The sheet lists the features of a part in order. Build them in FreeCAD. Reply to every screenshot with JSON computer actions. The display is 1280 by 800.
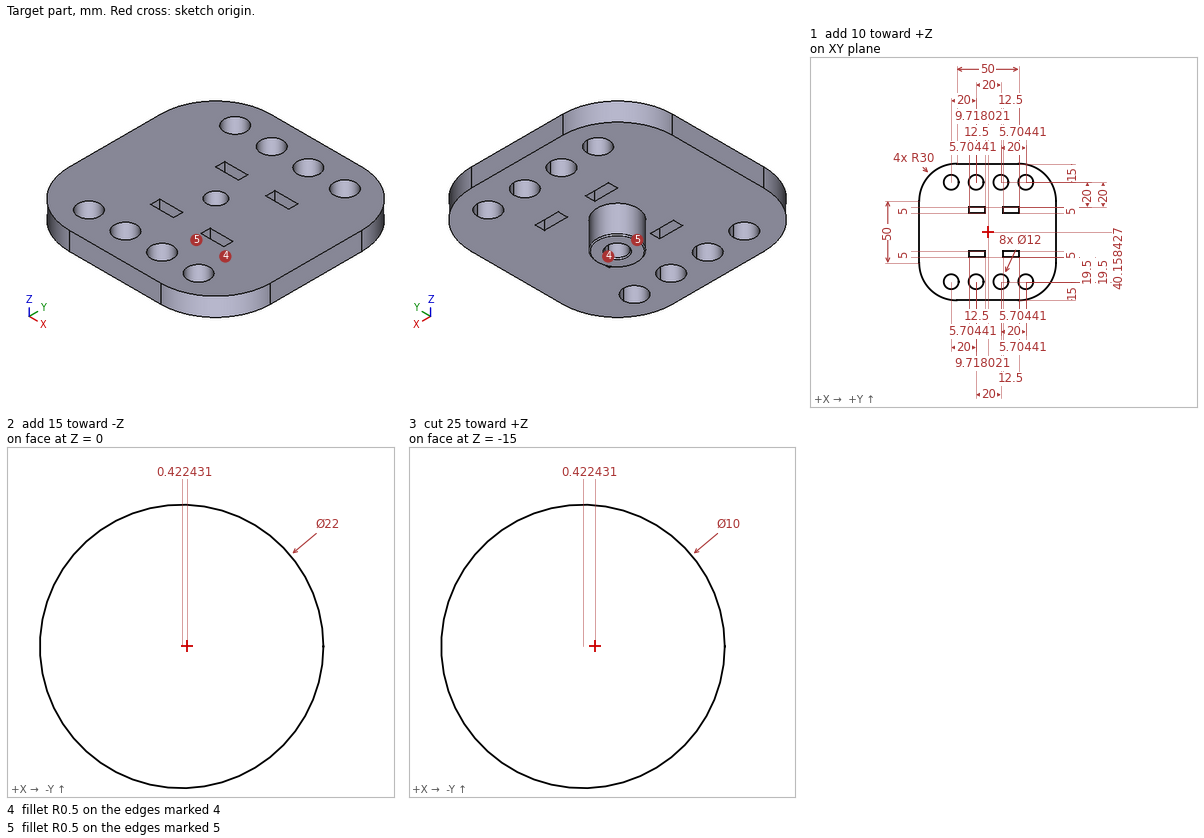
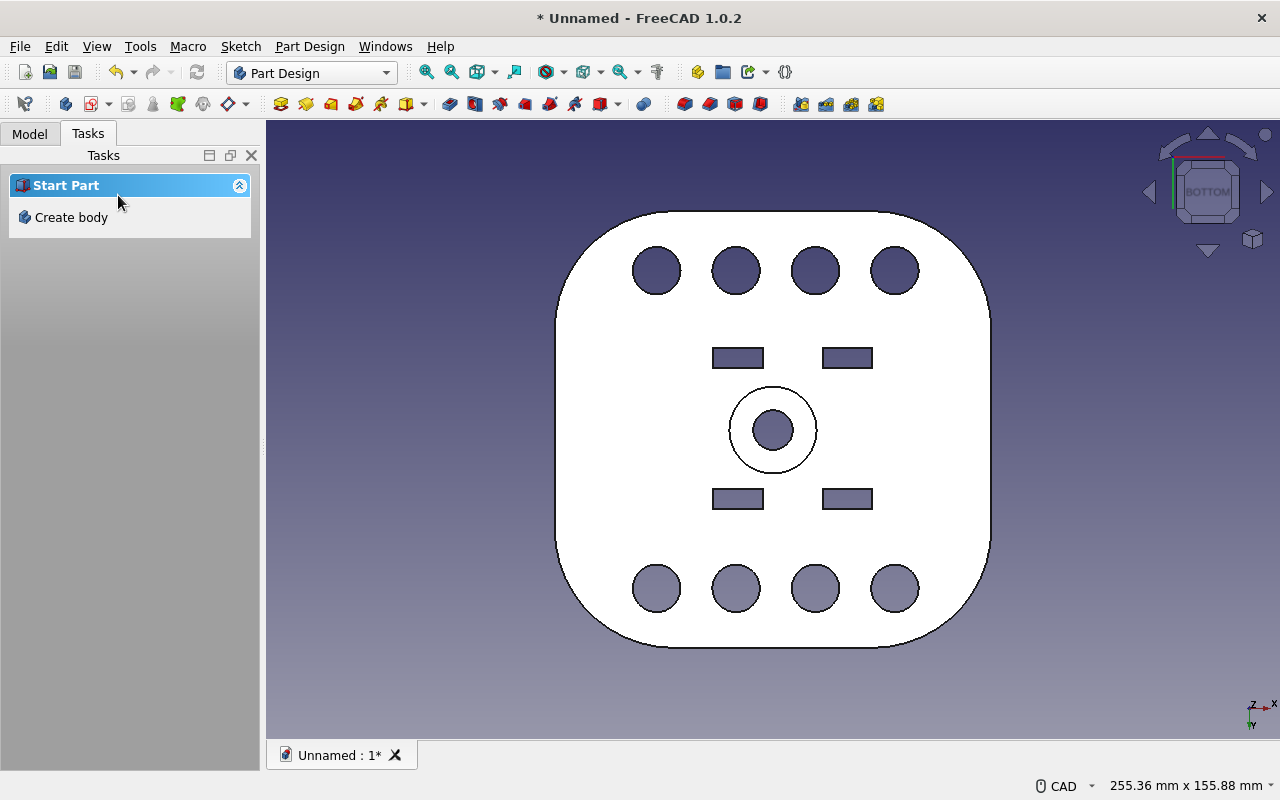
{"action": "left_click", "coordinate": [753, 429]}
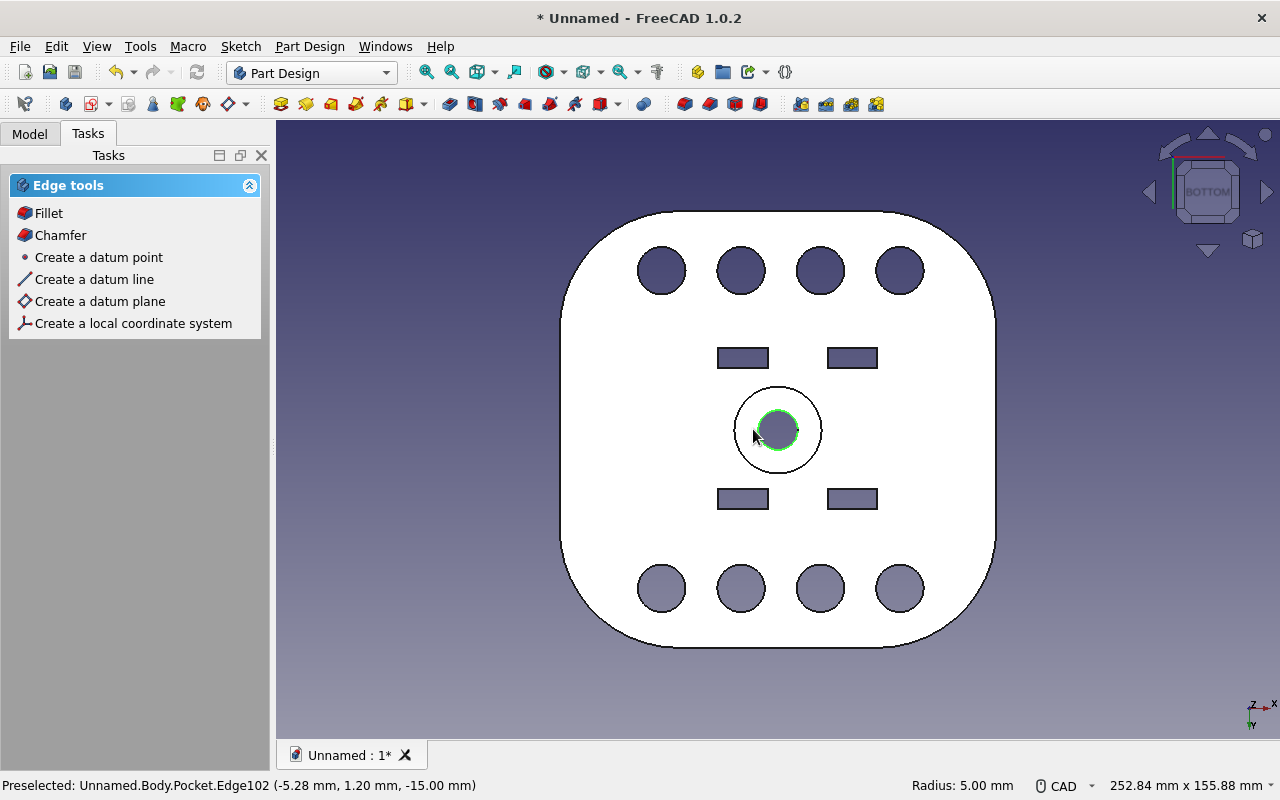
{"action": "left_click", "coordinate": [685, 104]}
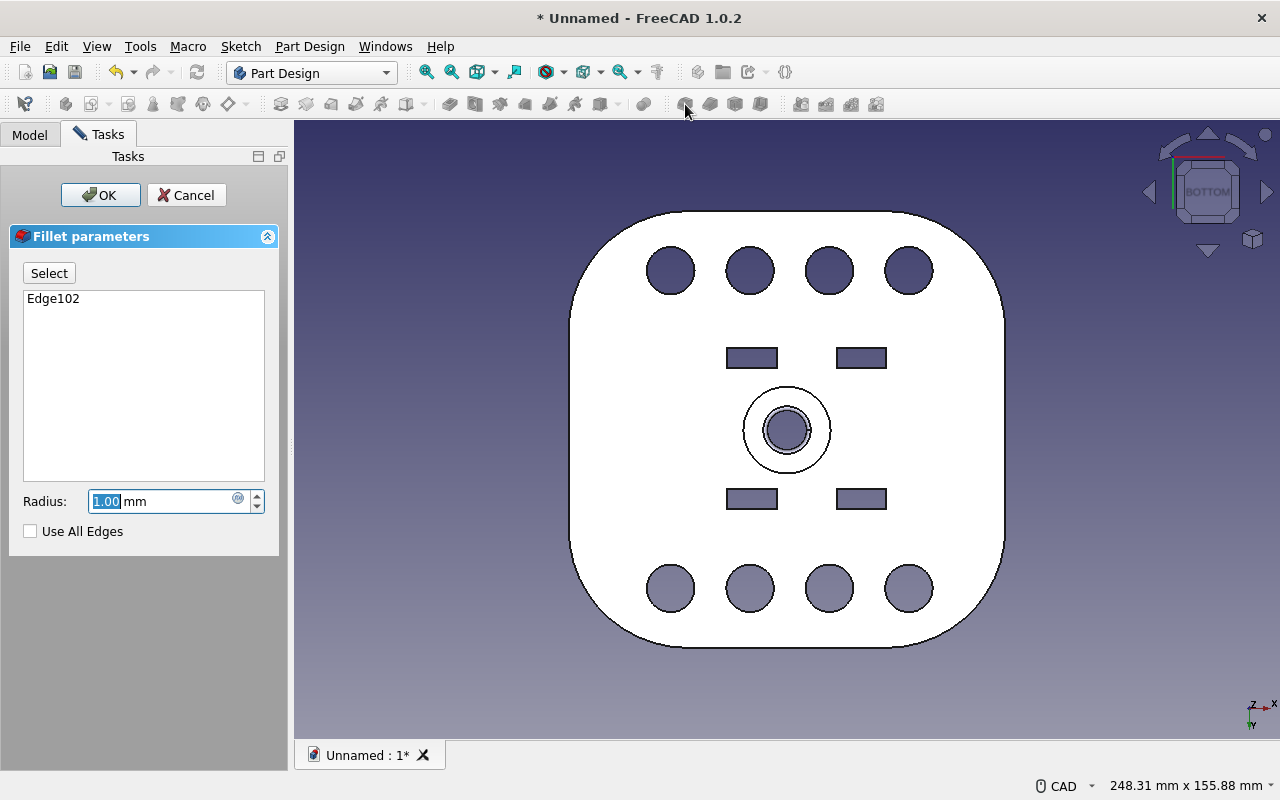
{"action": "type", "text": "0.5"}
{"action": "key", "text": "Tab"}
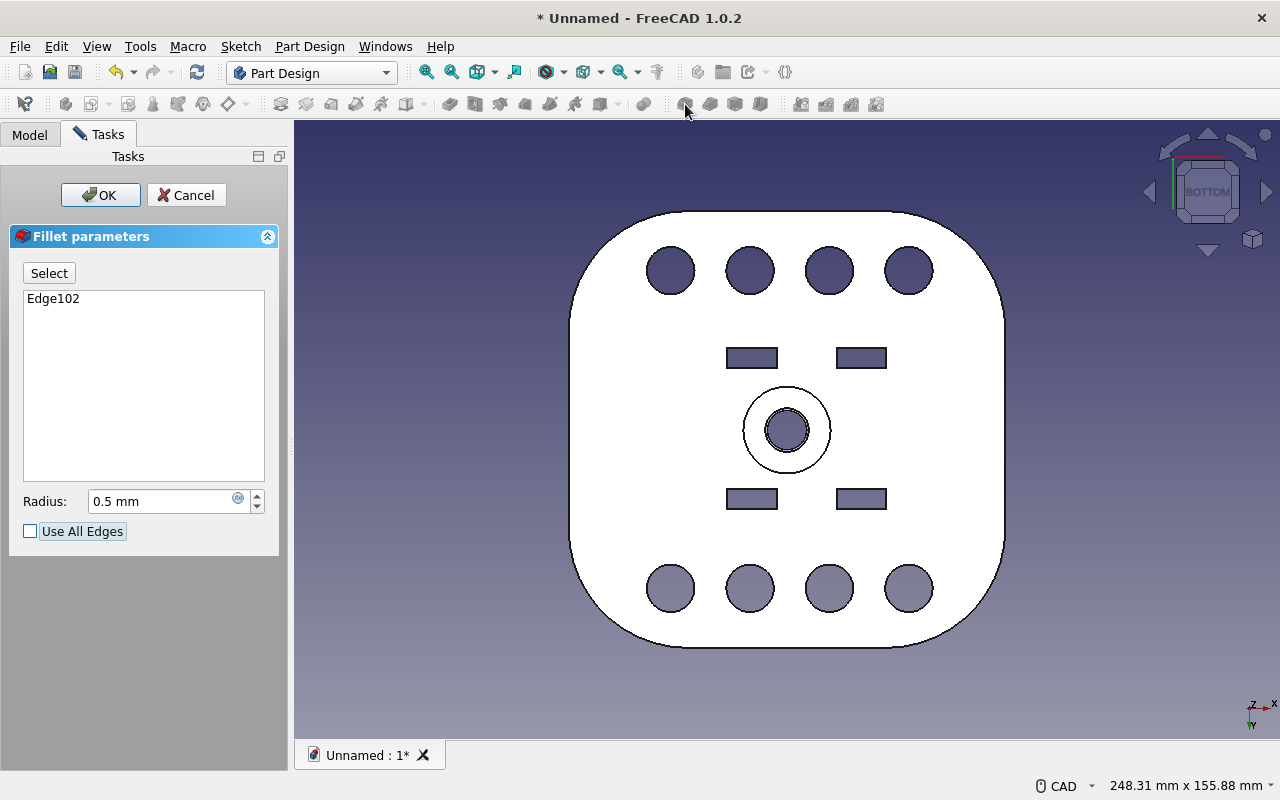
{"action": "left_click", "coordinate": [101, 195]}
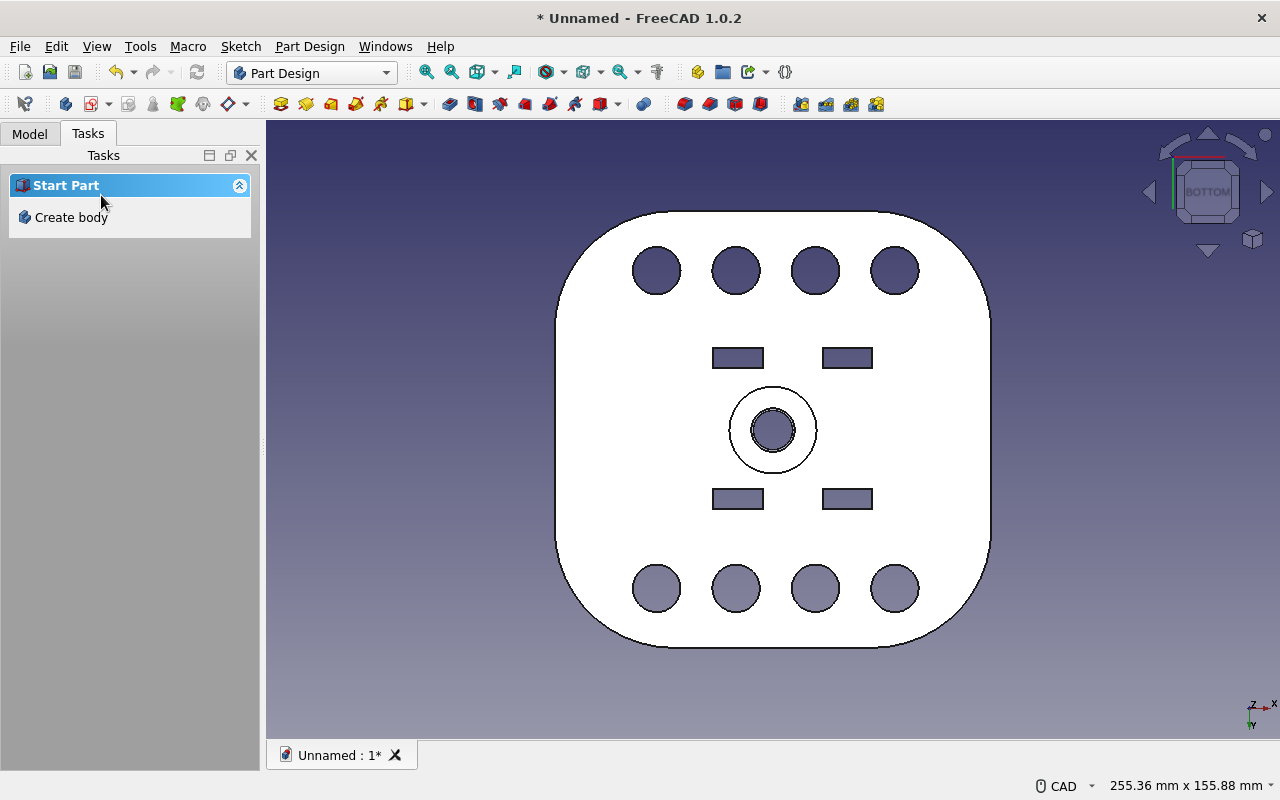
{"action": "left_click", "coordinate": [729, 429]}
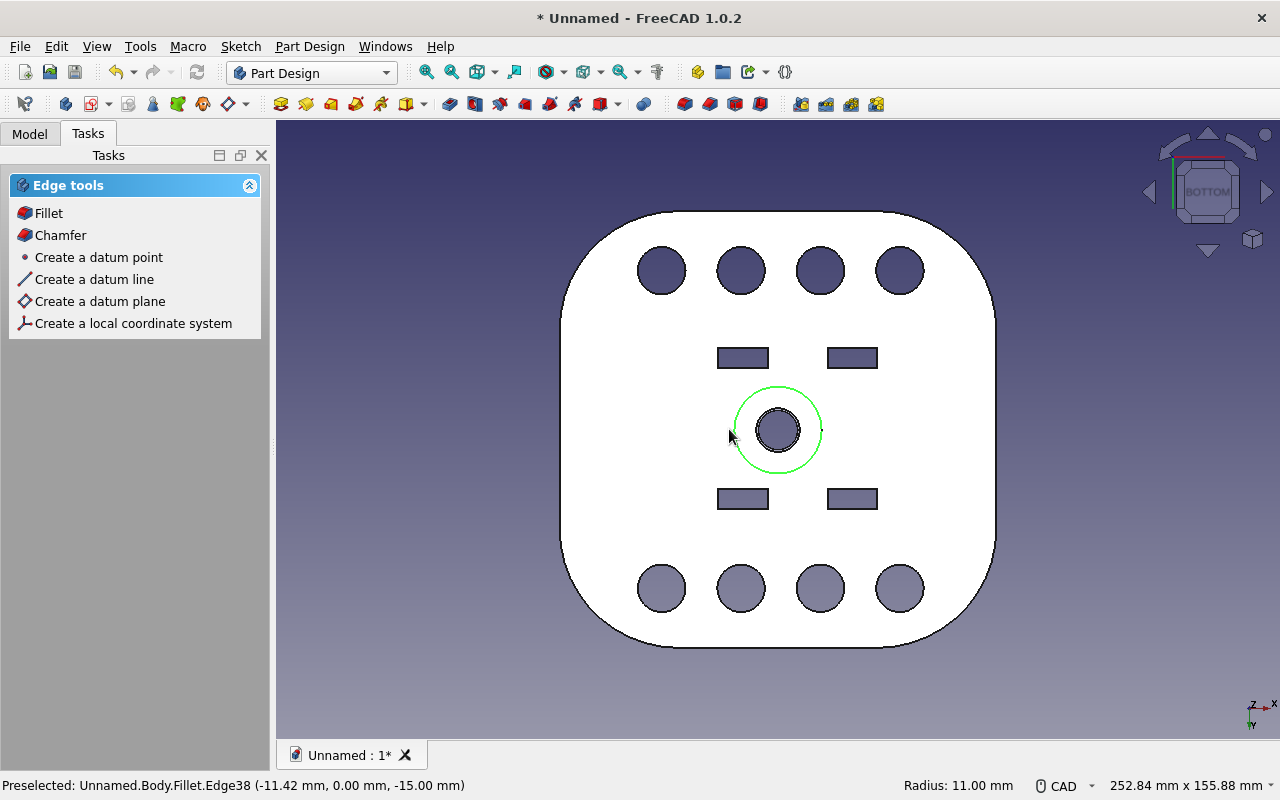
{"action": "left_click", "coordinate": [685, 104]}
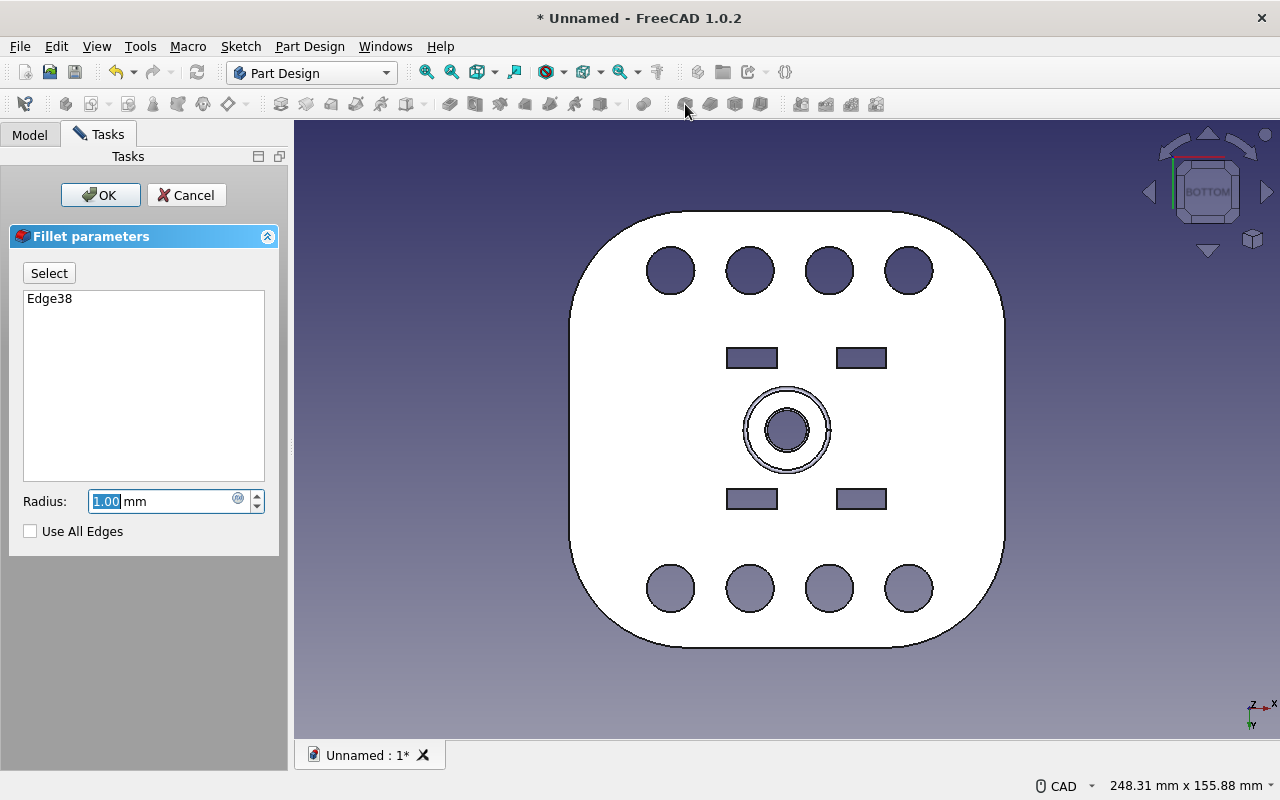
{"action": "type", "text": "0.5"}
{"action": "key", "text": "Tab"}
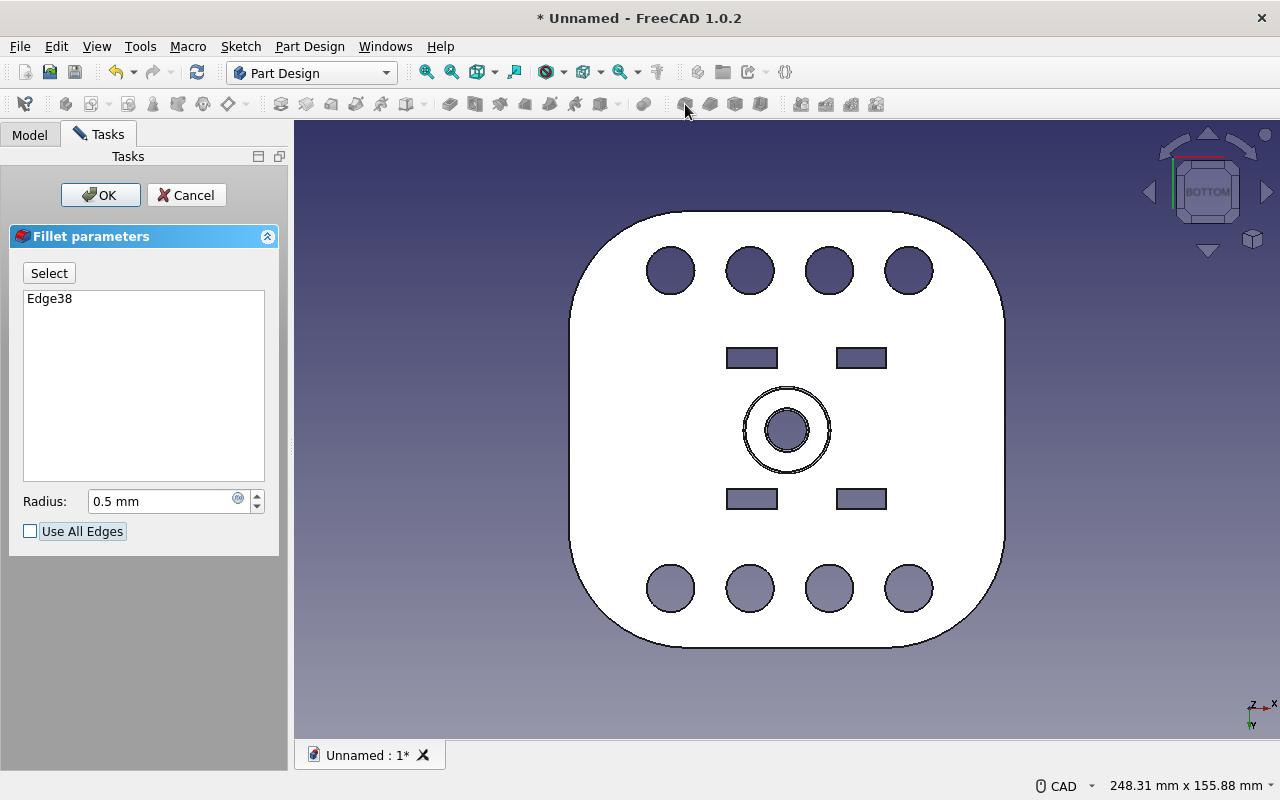
{"action": "left_click", "coordinate": [101, 195]}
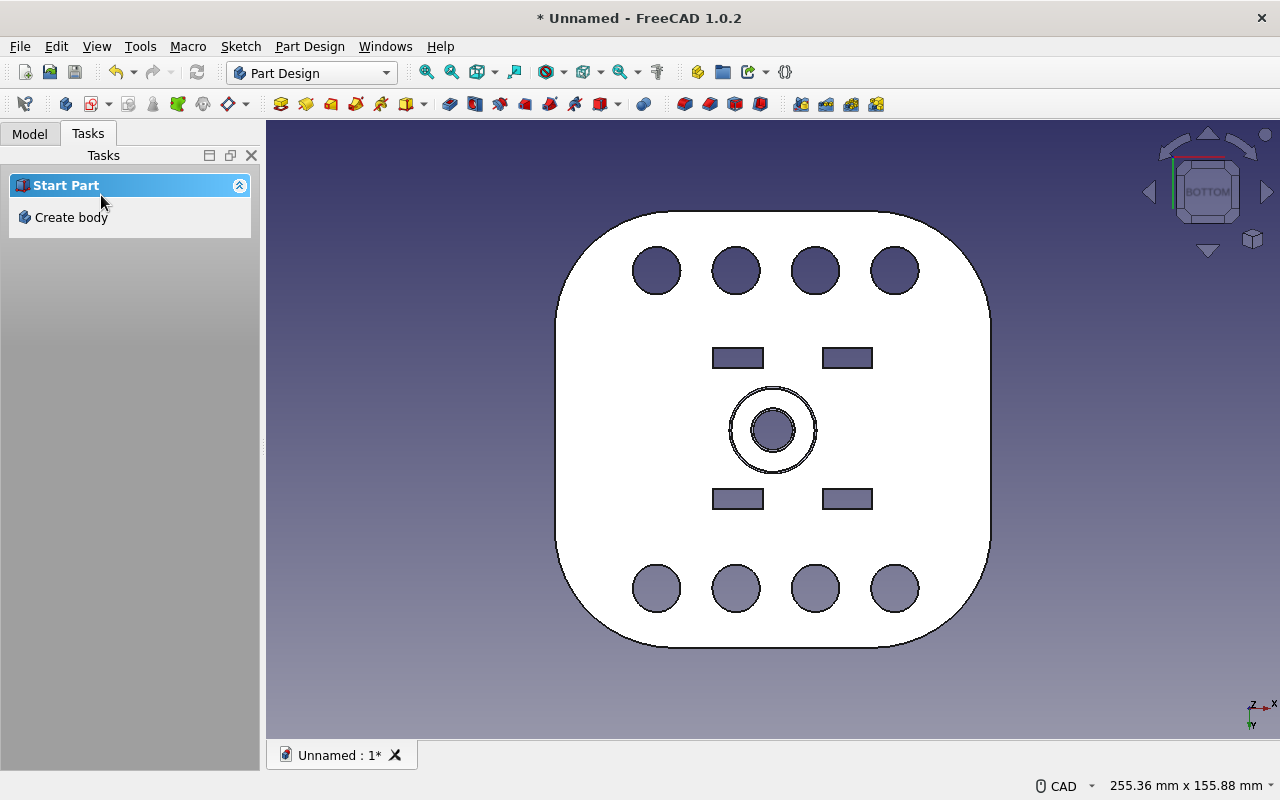
{"action": "key", "text": "0"}